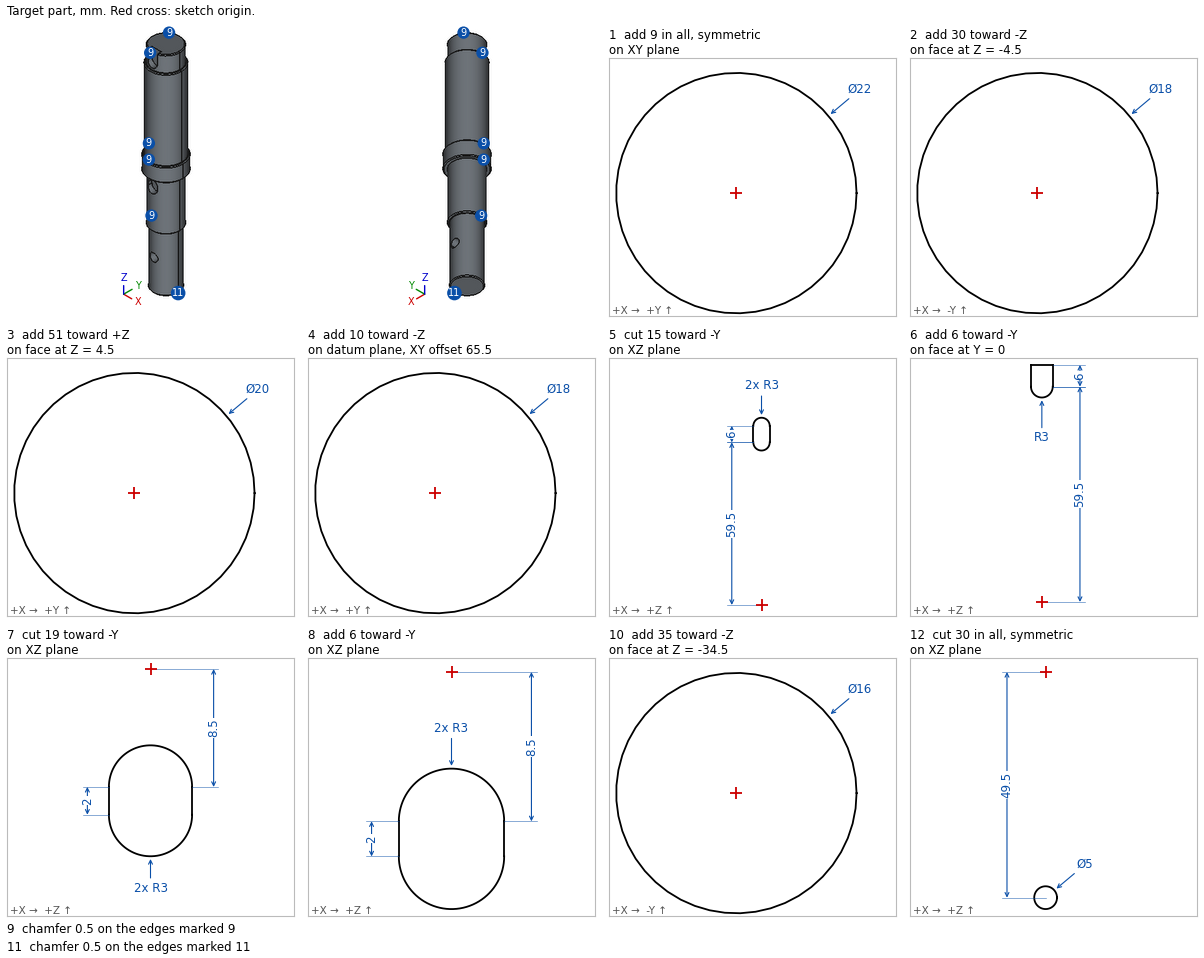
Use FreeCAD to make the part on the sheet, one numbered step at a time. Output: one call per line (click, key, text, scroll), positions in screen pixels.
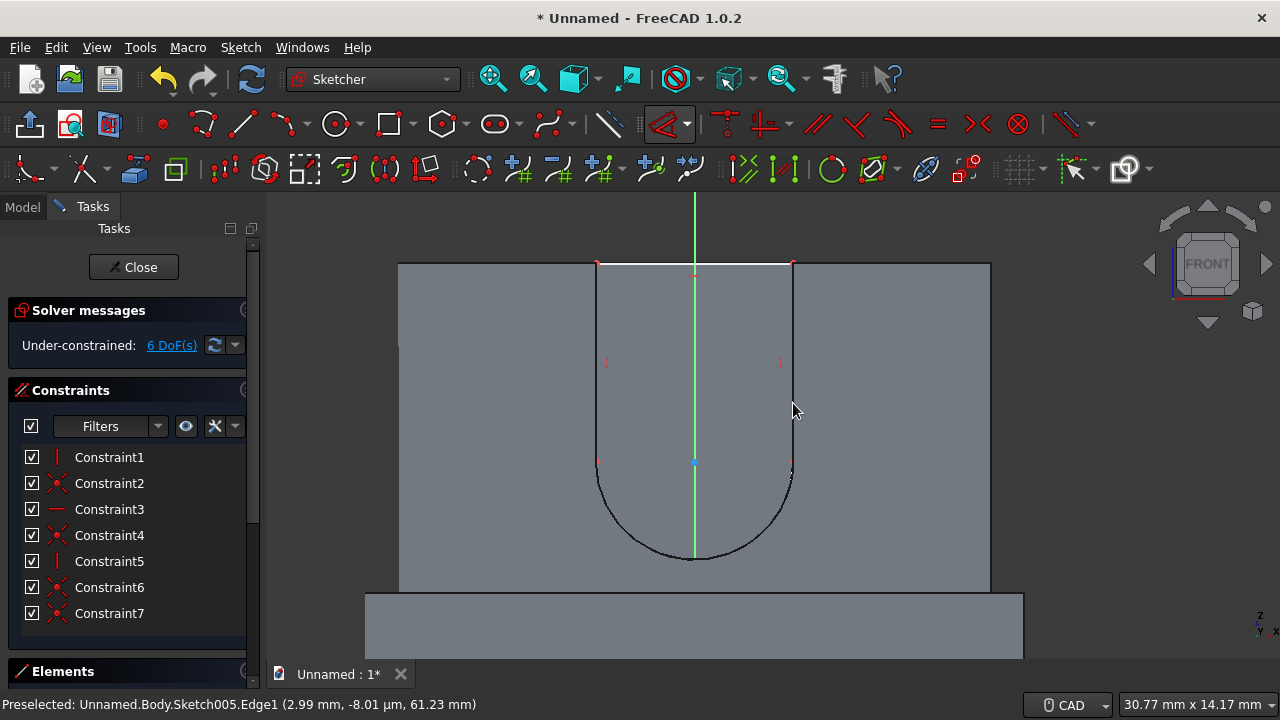
click(636, 542)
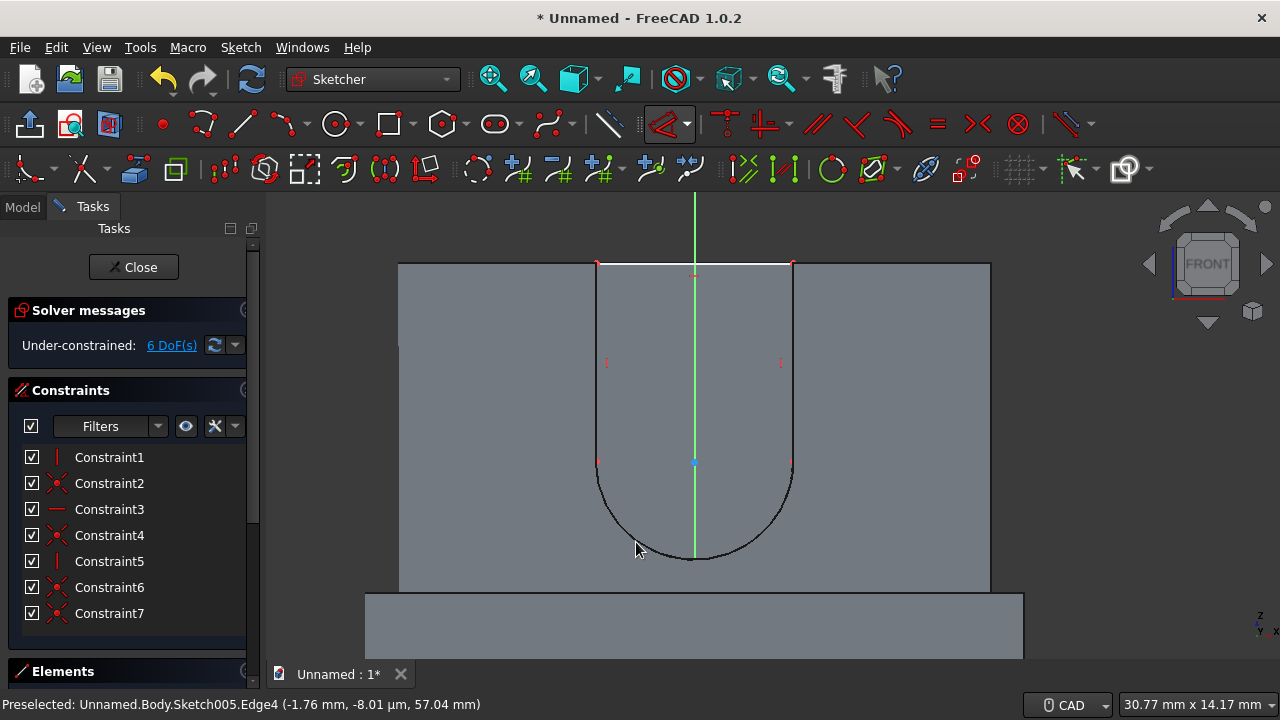
click(898, 124)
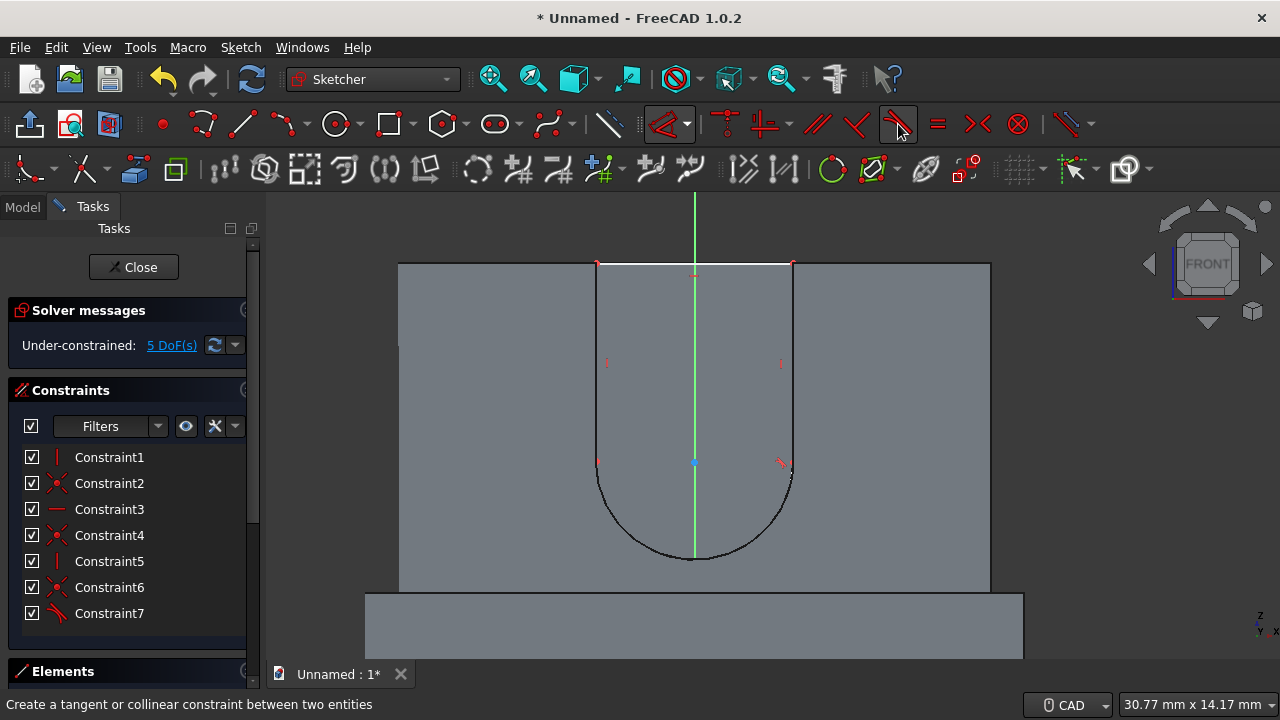
click(596, 323)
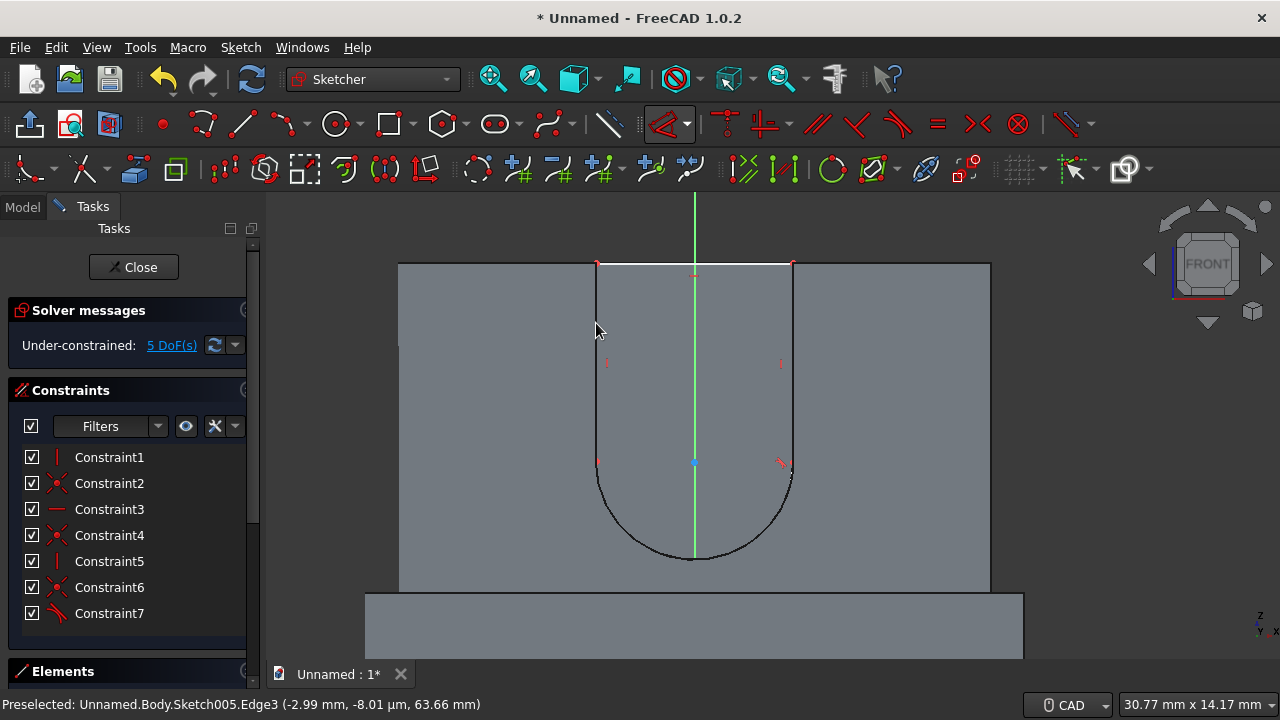
click(636, 542)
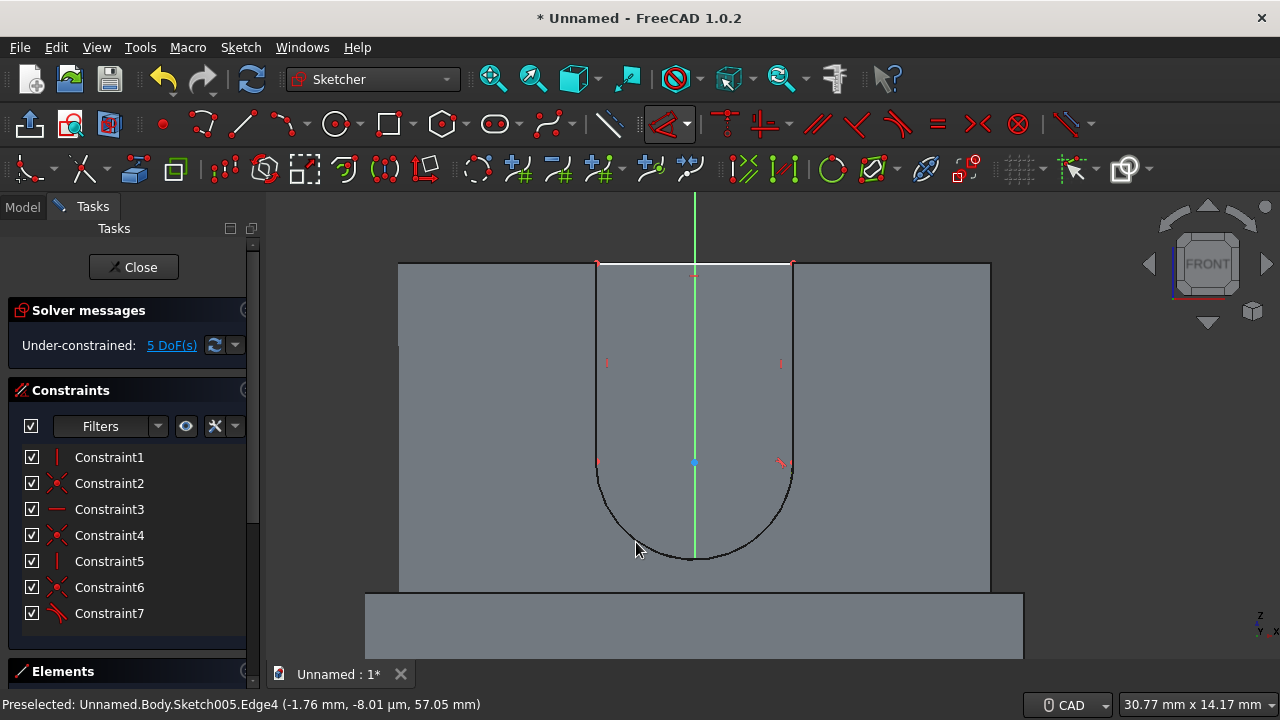
click(898, 124)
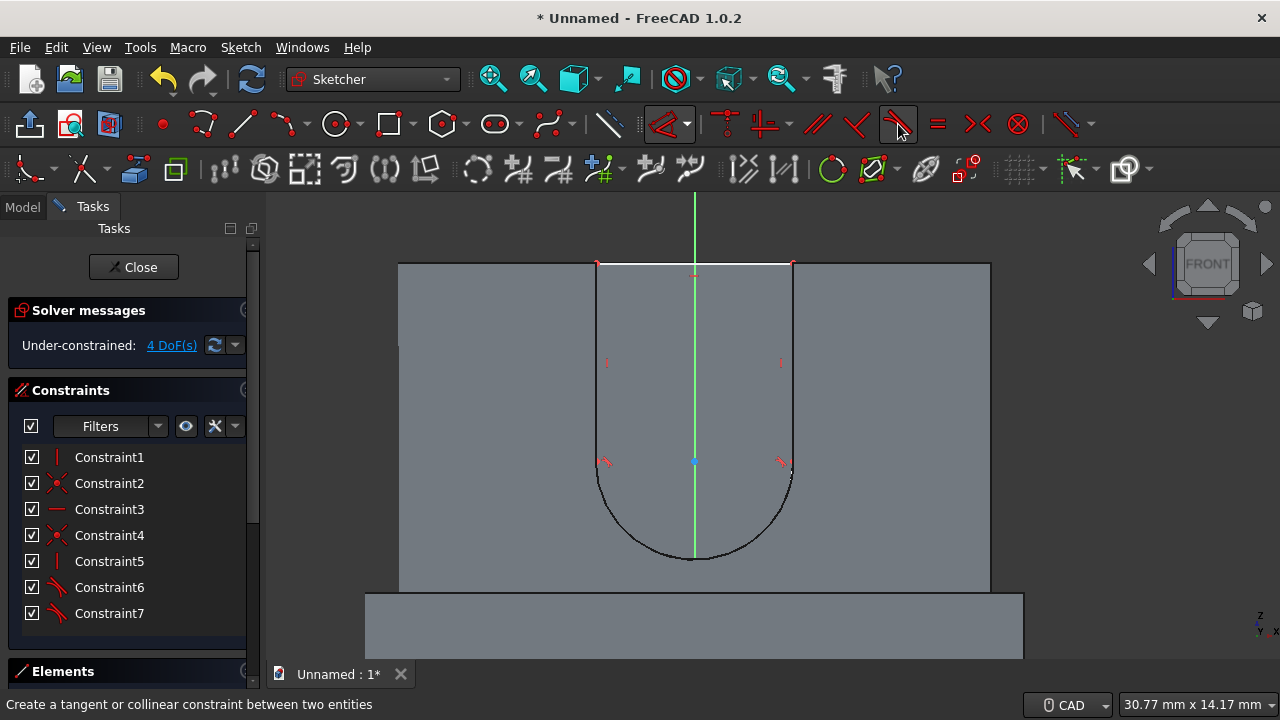
click(695, 462)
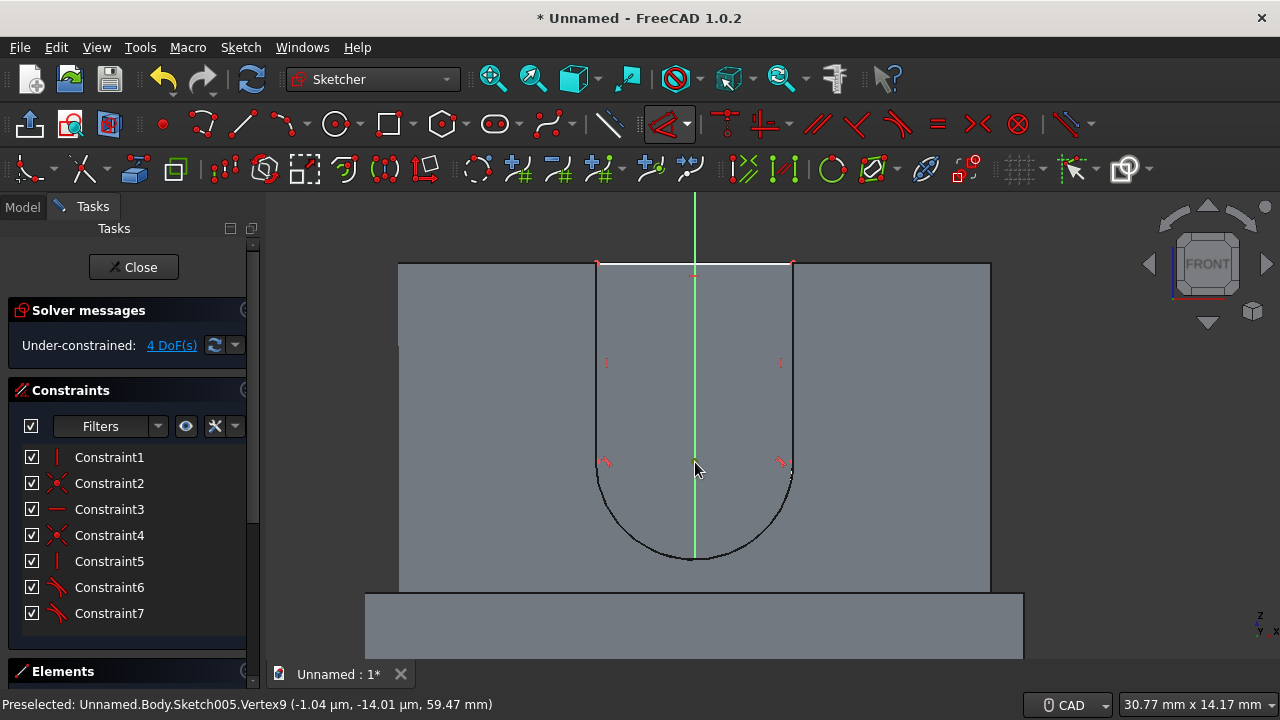
click(695, 602)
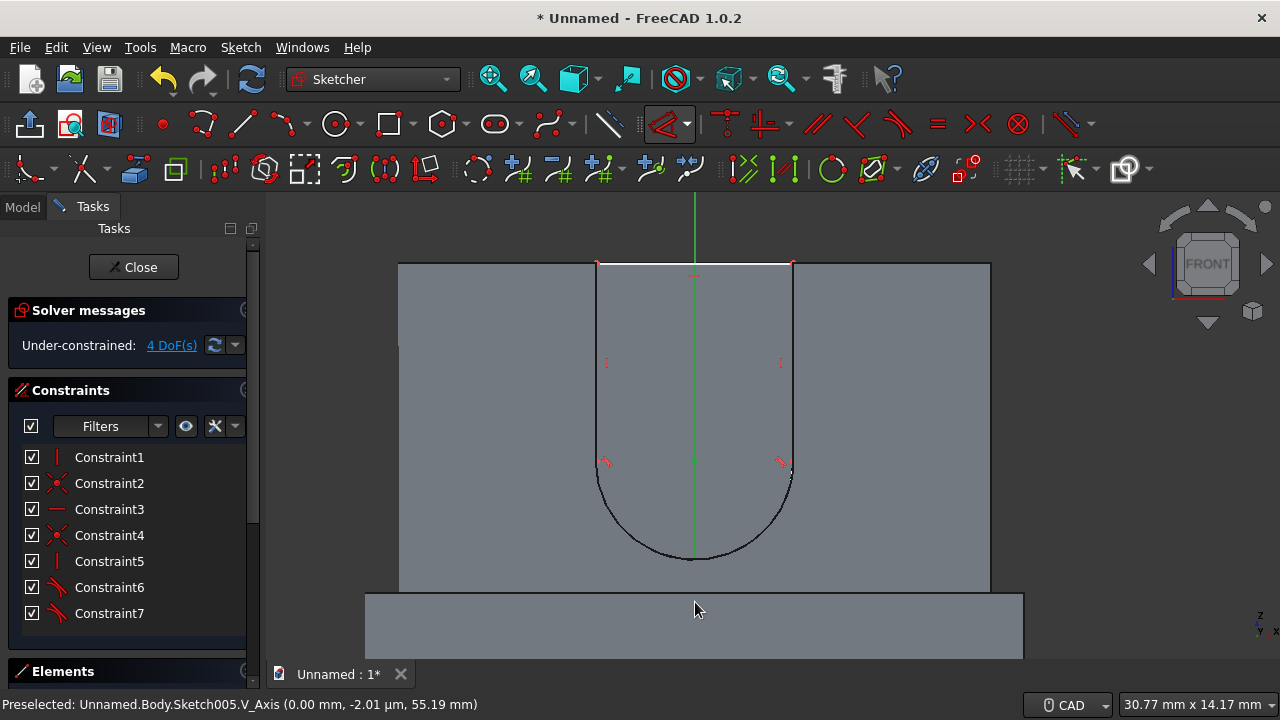
click(726, 124)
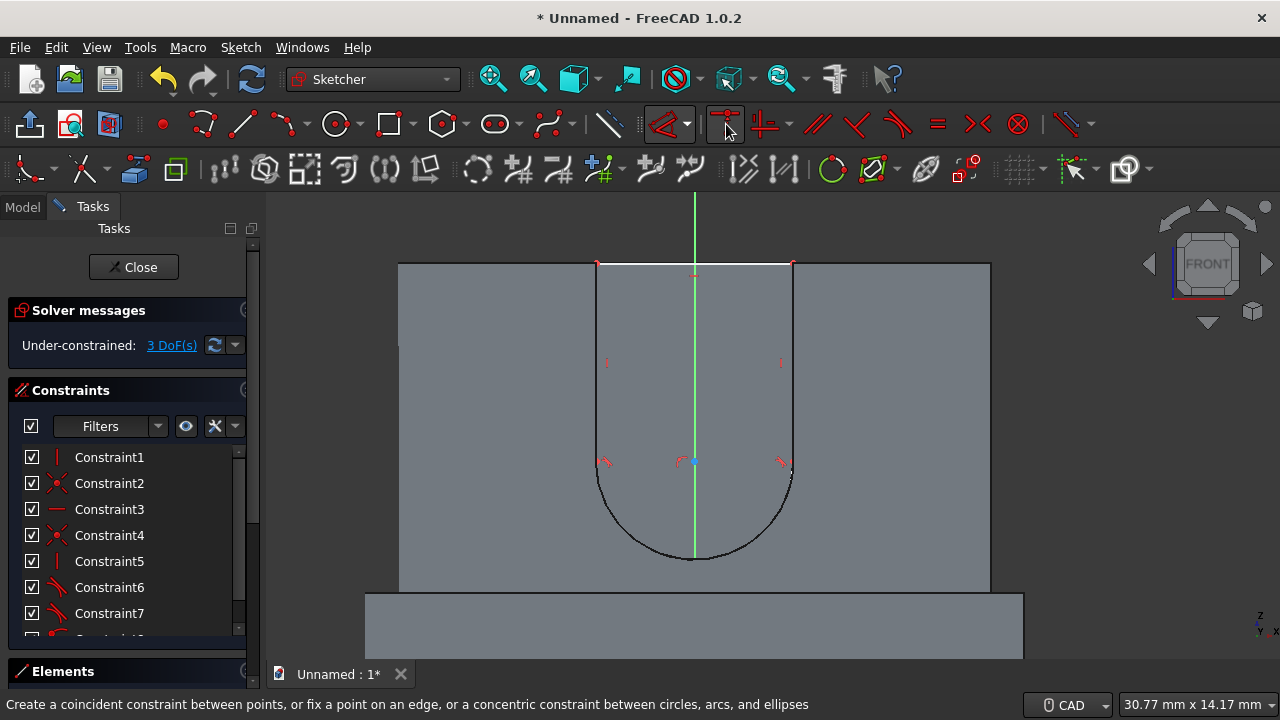
click(637, 542)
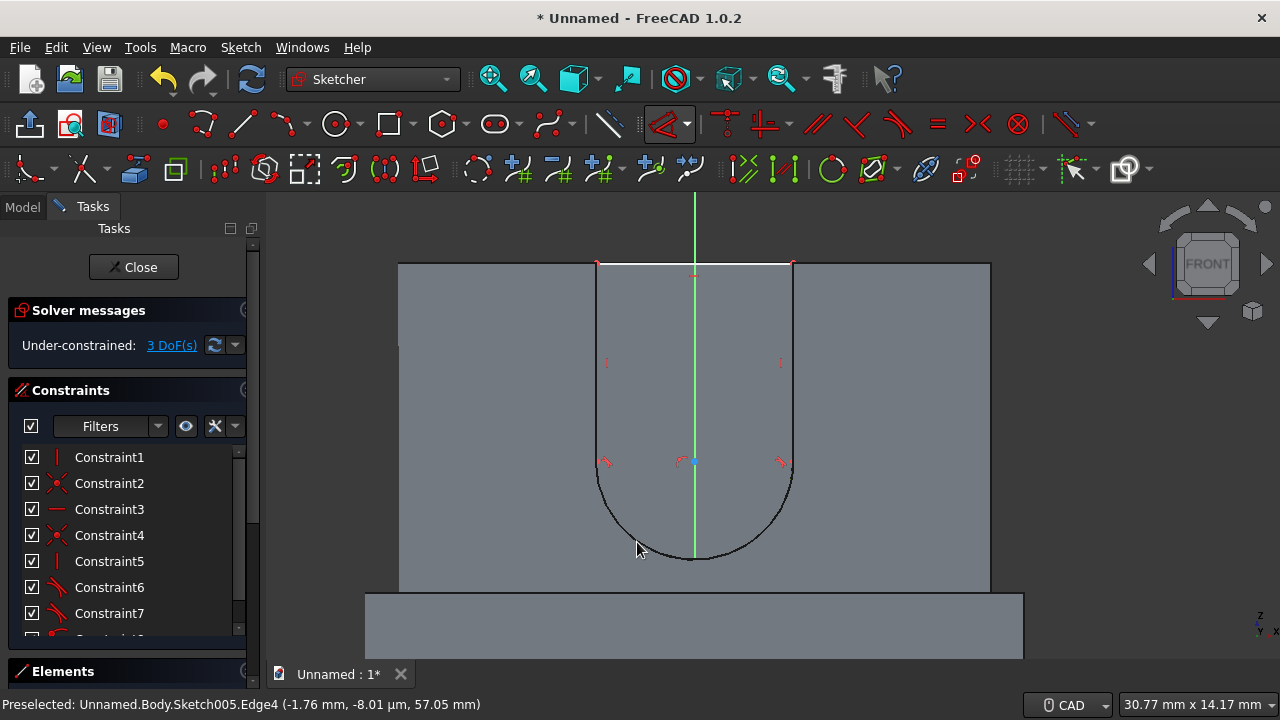
click(690, 124)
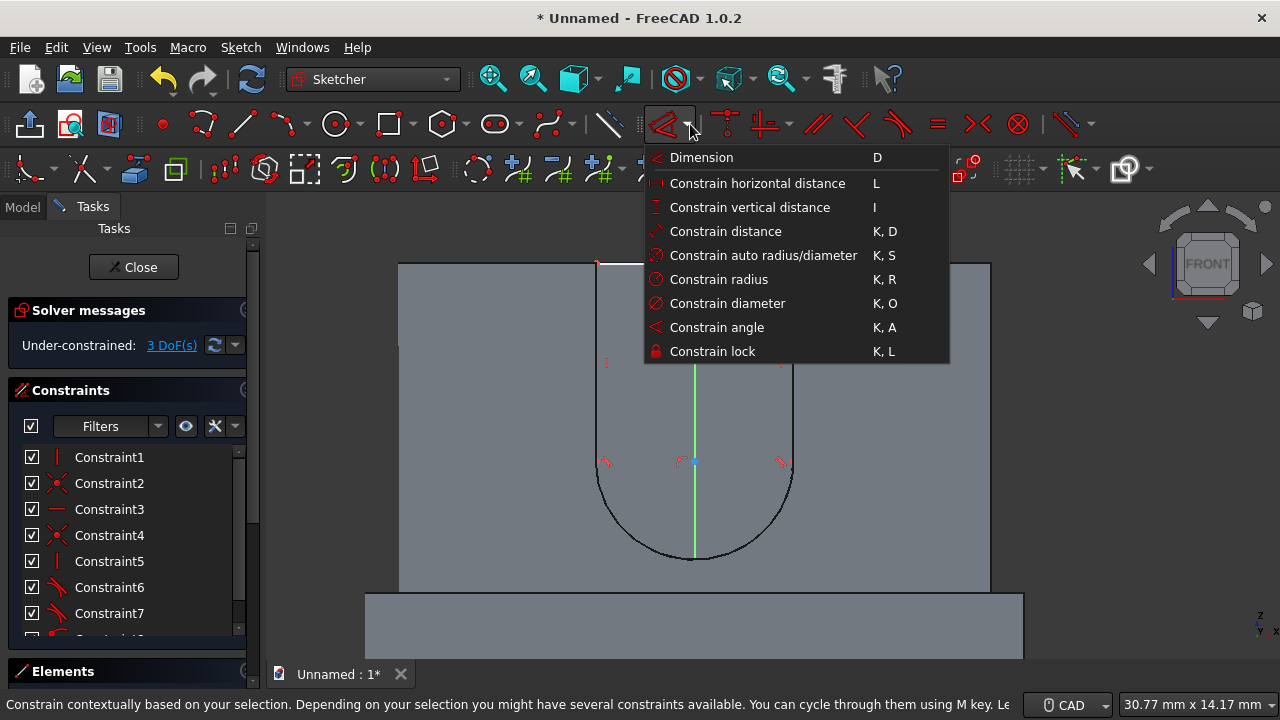
click(797, 279)